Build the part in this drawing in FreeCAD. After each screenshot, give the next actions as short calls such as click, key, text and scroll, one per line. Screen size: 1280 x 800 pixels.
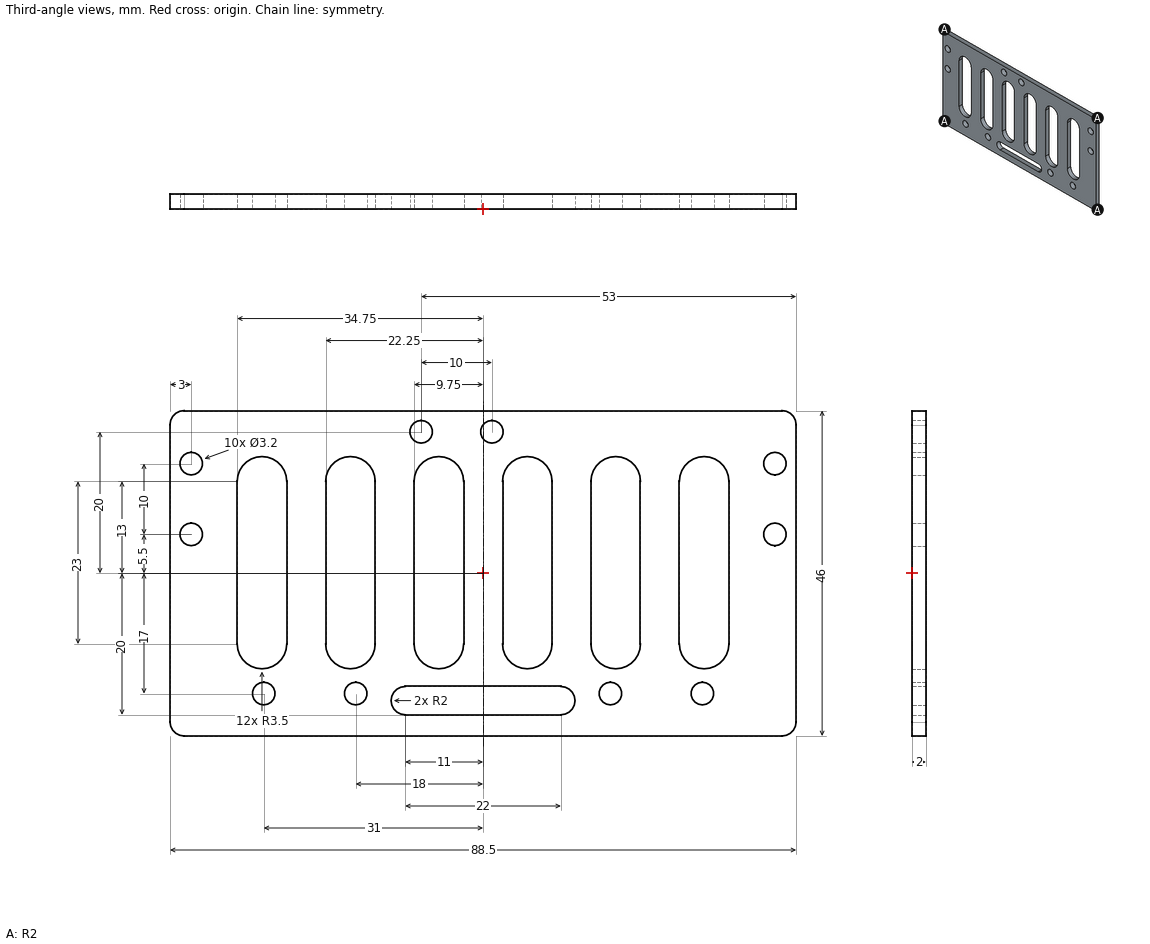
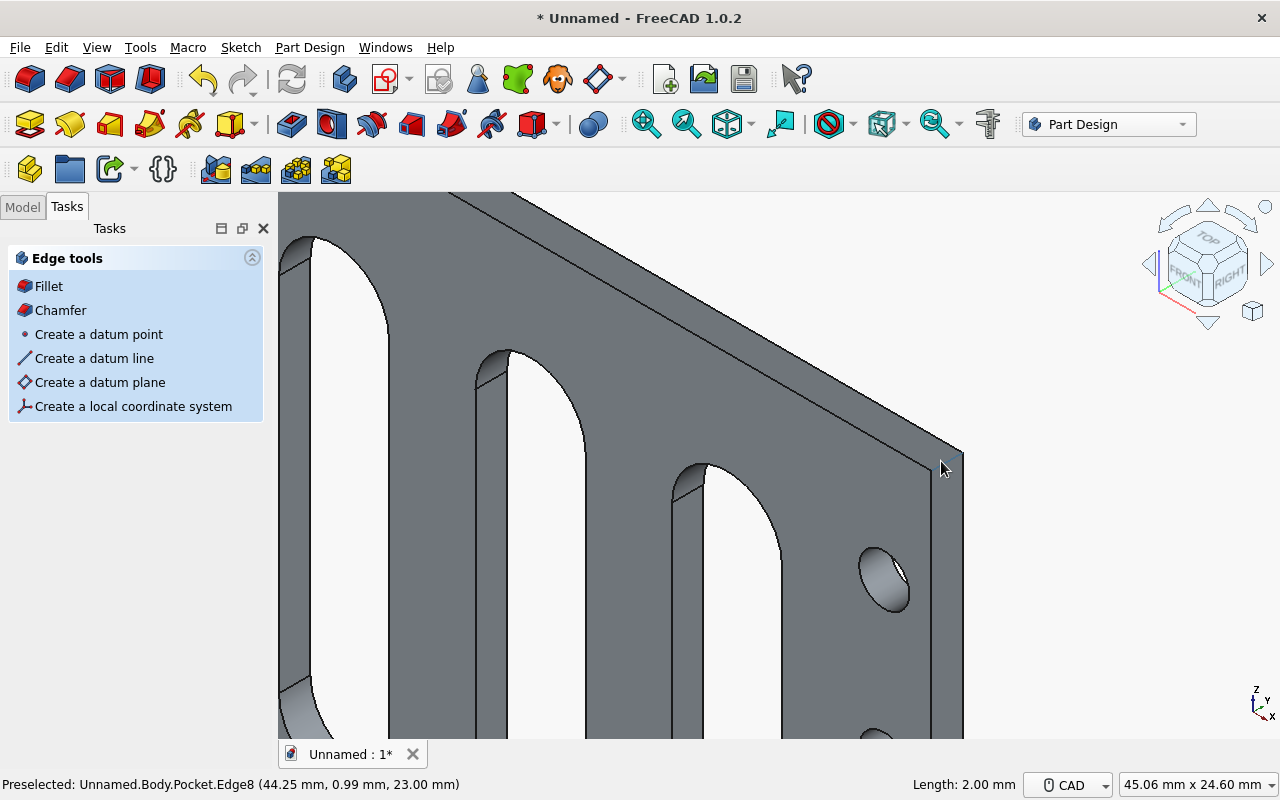
click(648, 124)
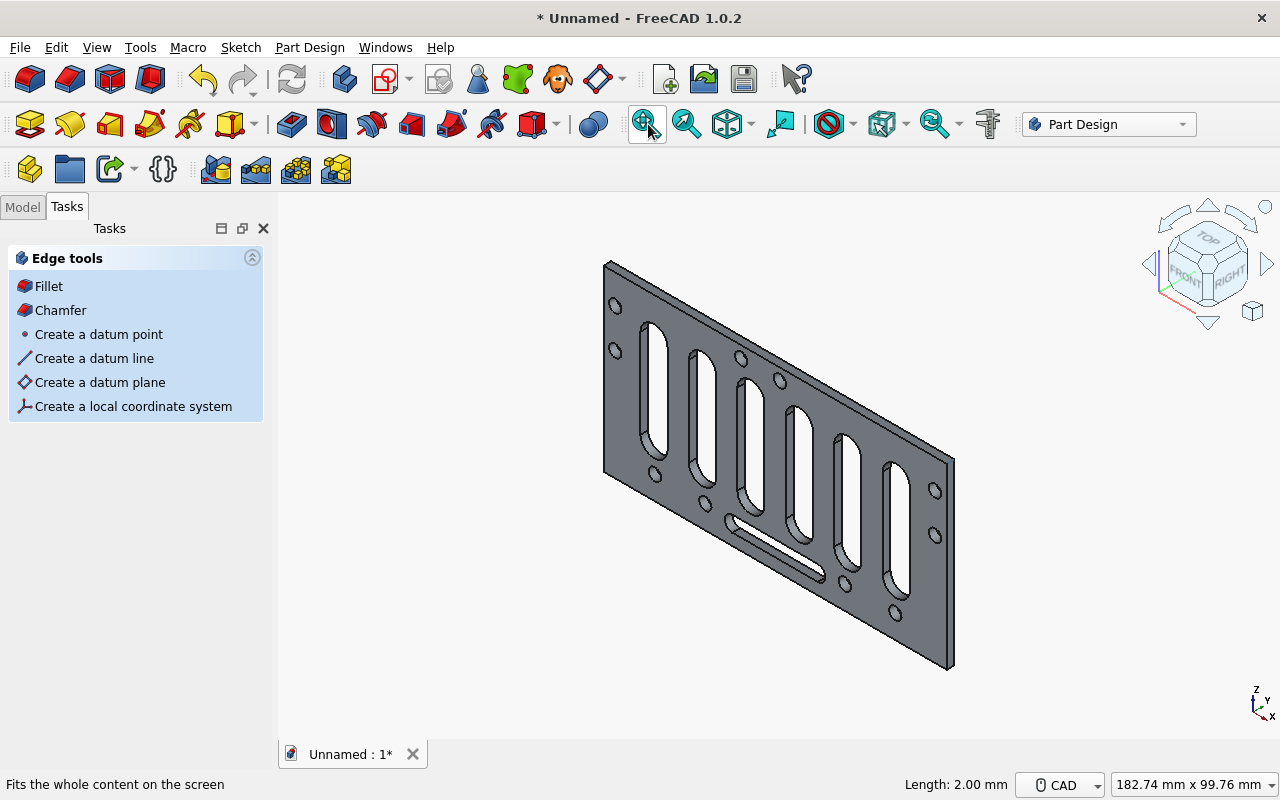
key(2)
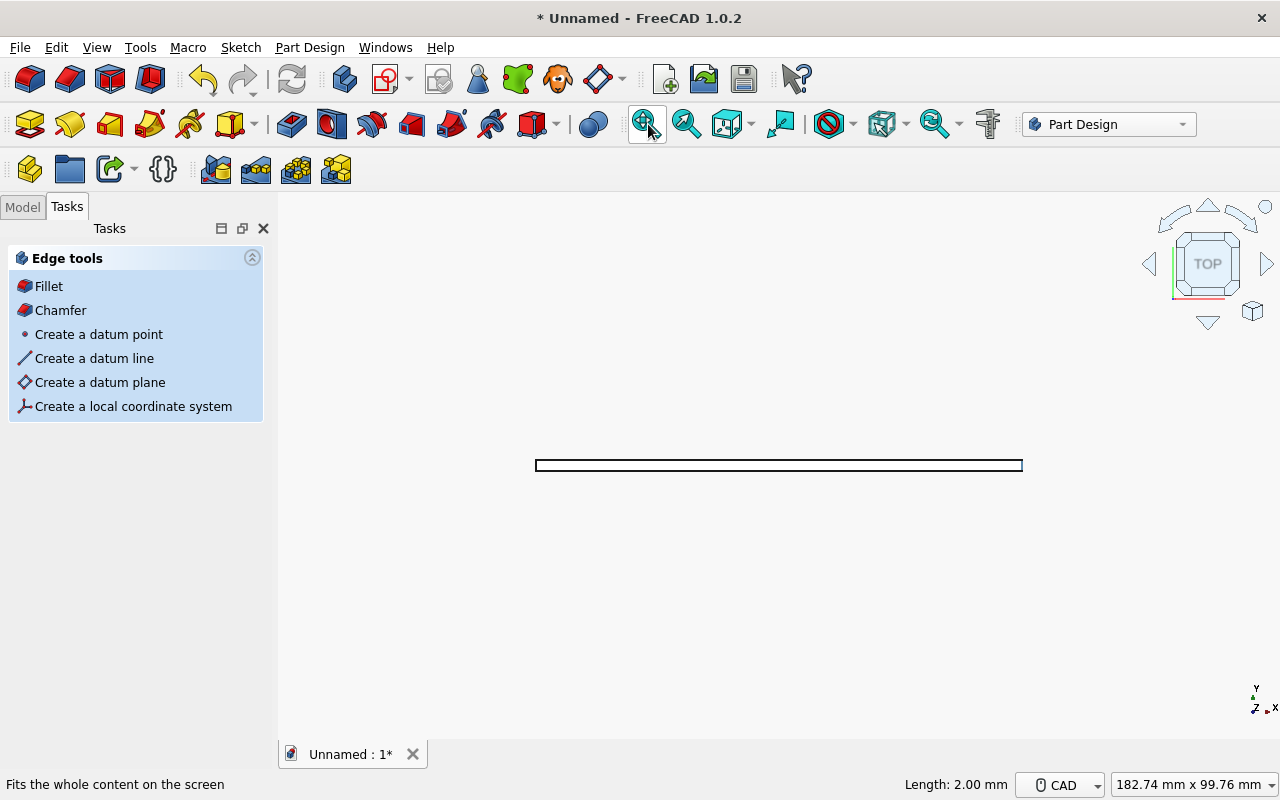
click(536, 466, ctrl)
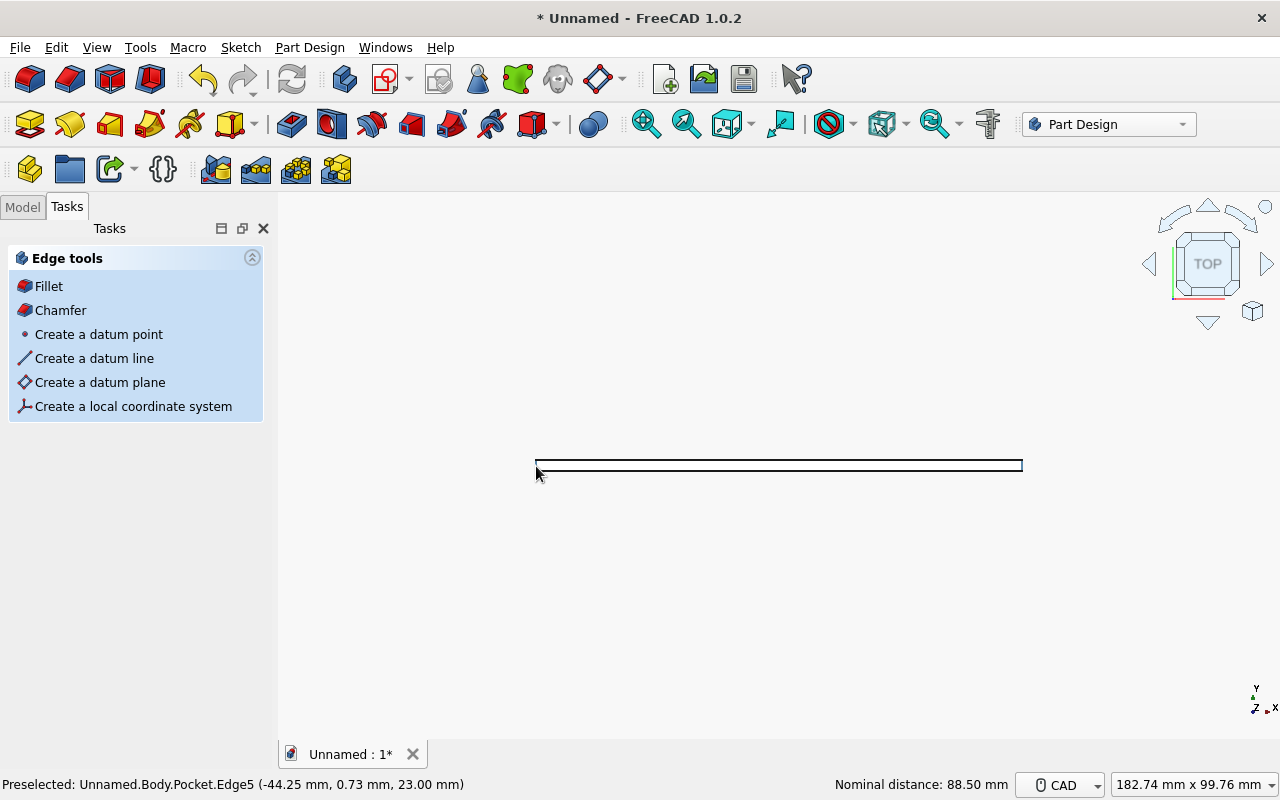
scroll(536, 464, up, 7)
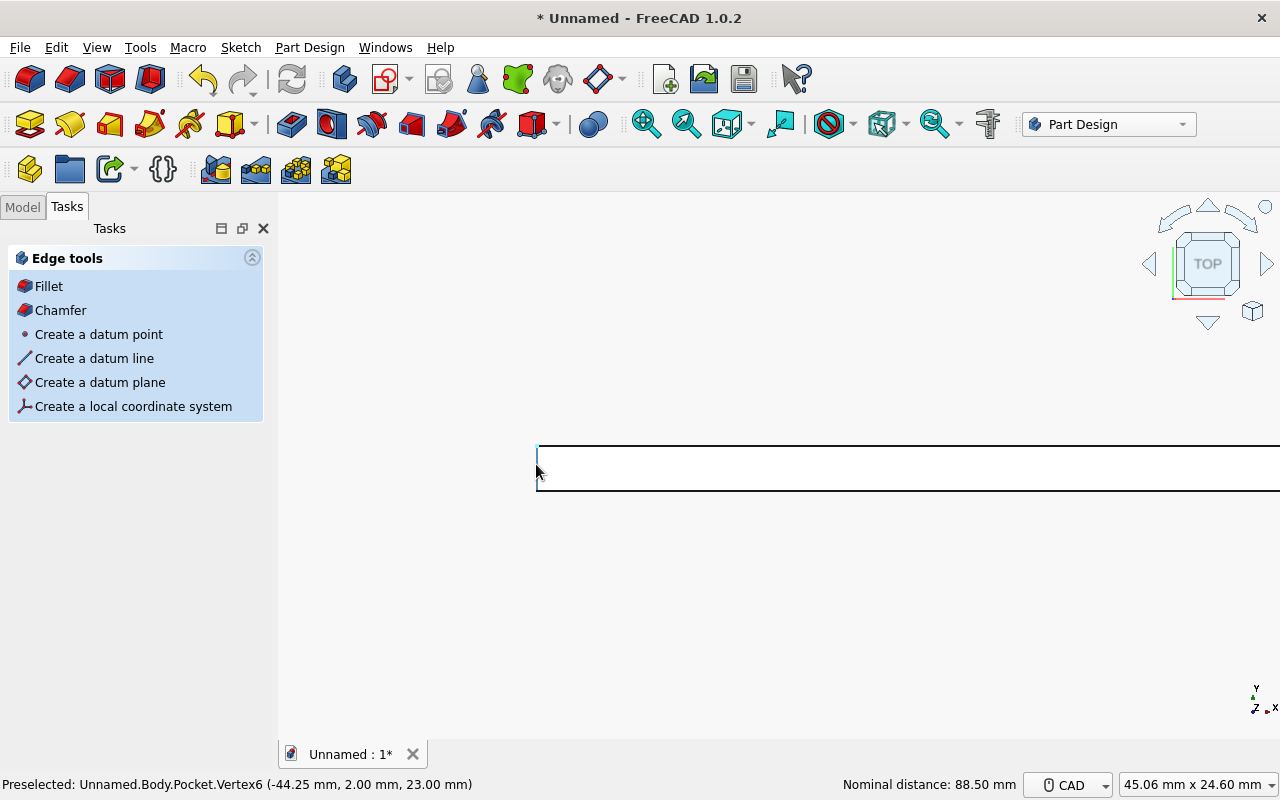
click(648, 124)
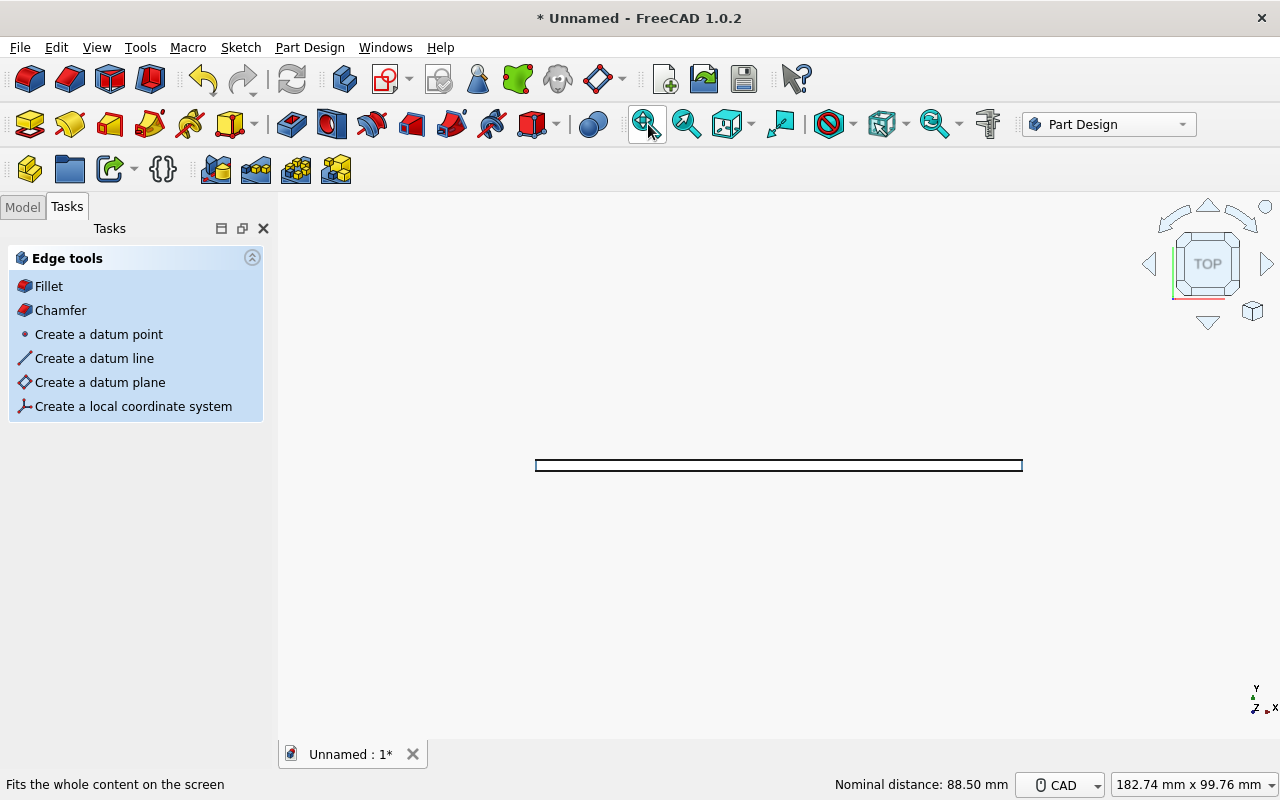
key(1)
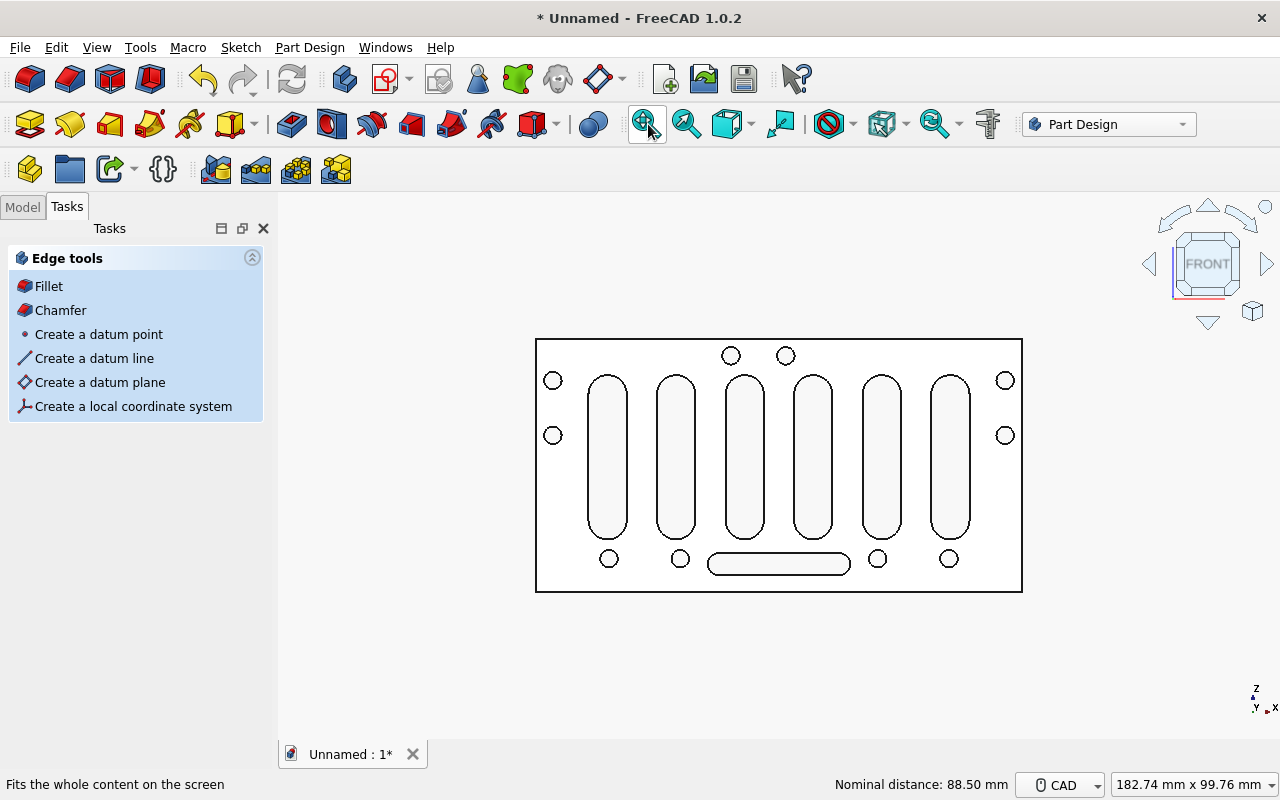
scroll(536, 591, up, 7)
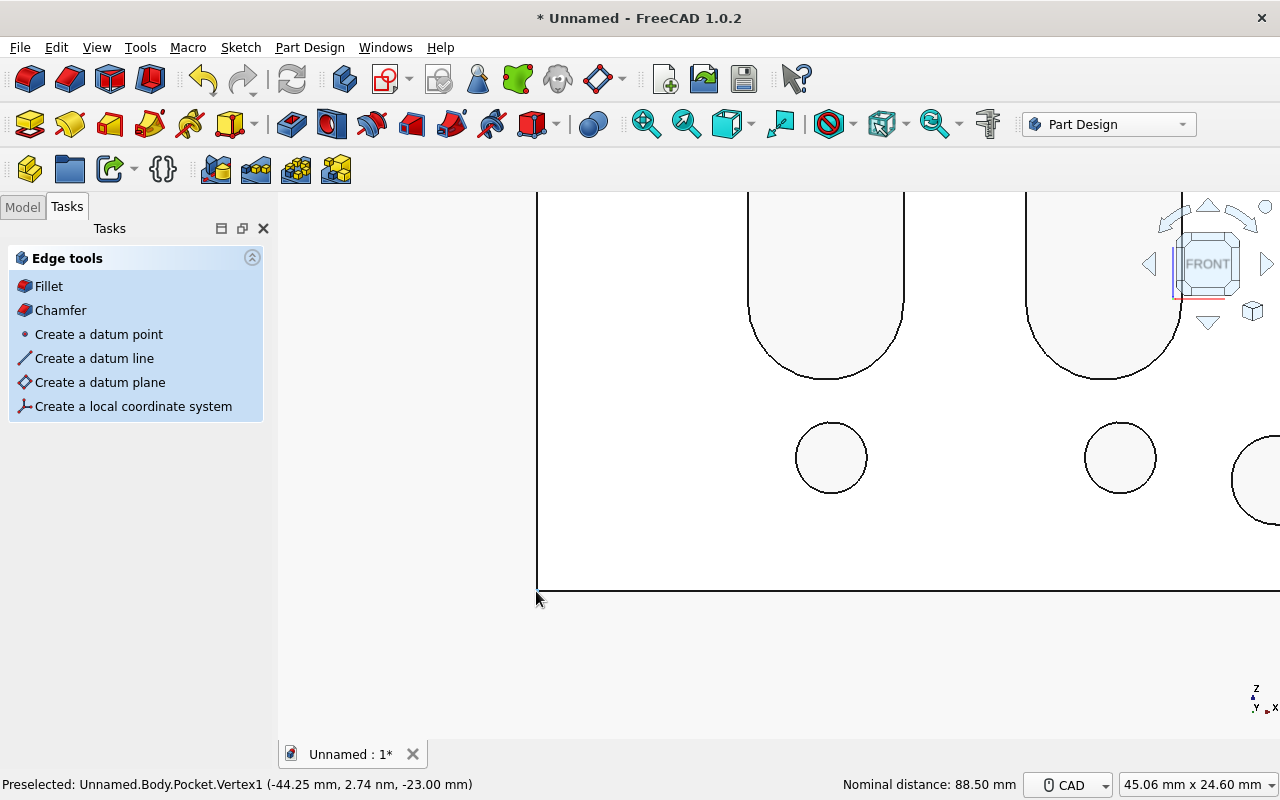
click(648, 124)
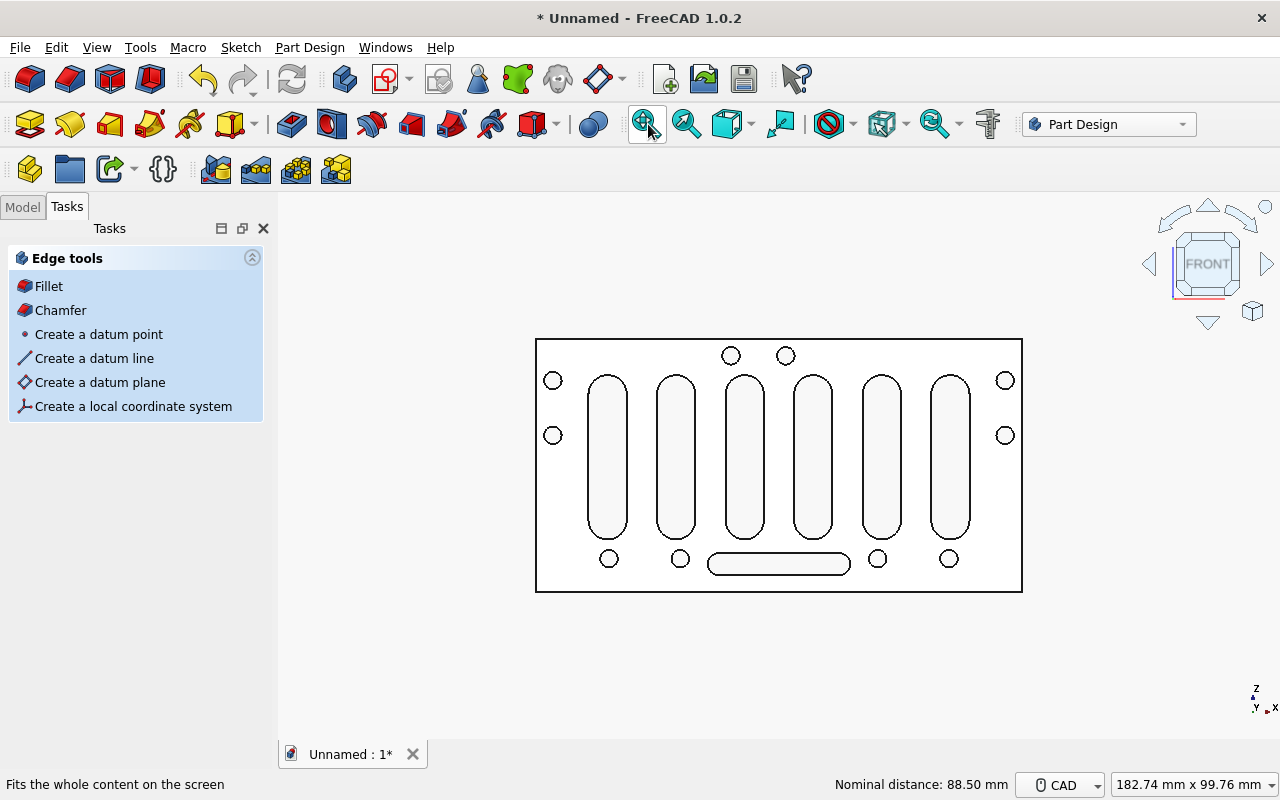
key(3)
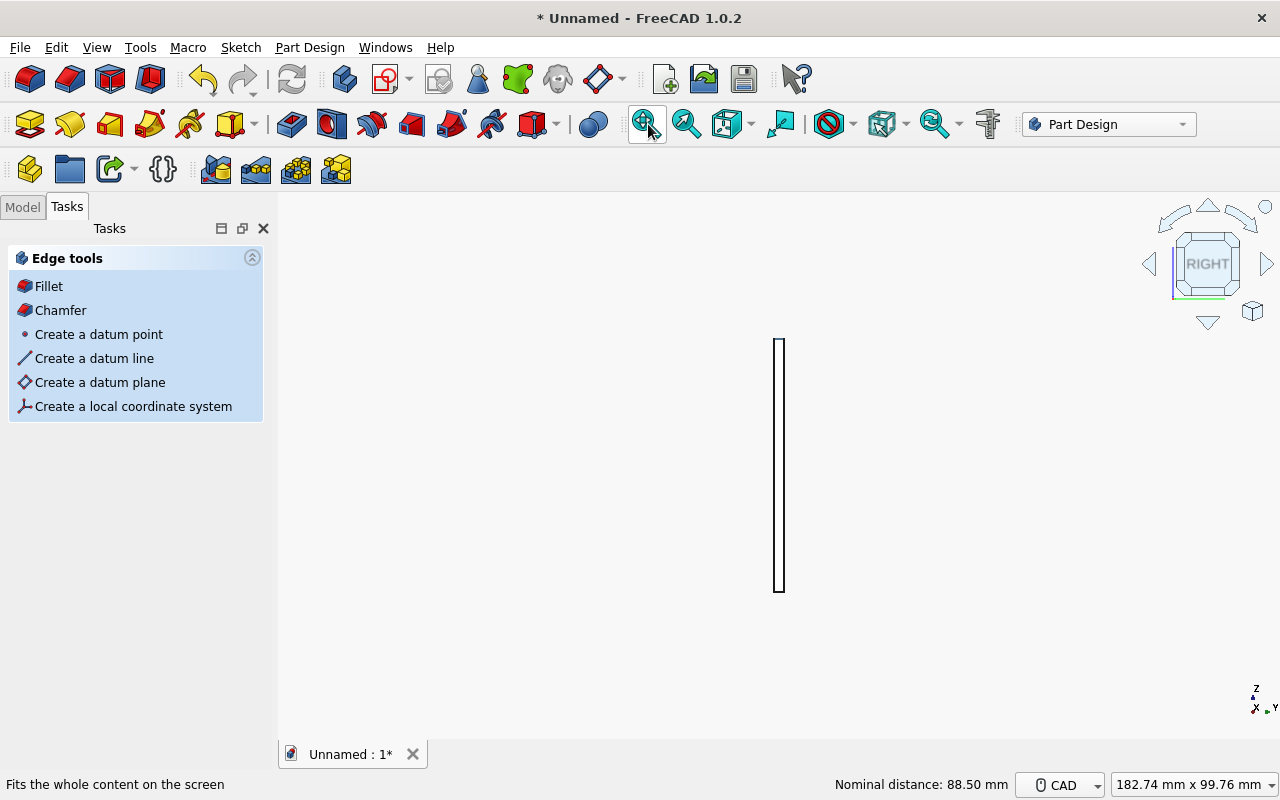
scroll(779, 591, up, 7)